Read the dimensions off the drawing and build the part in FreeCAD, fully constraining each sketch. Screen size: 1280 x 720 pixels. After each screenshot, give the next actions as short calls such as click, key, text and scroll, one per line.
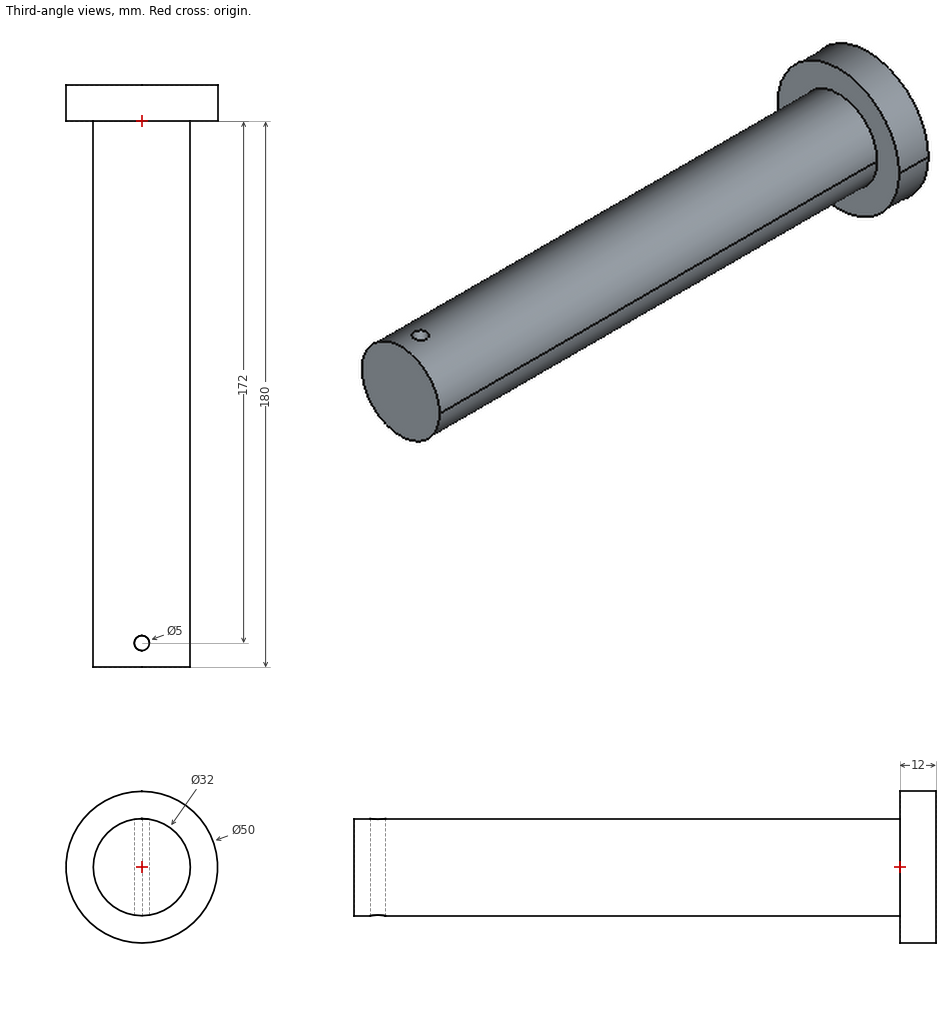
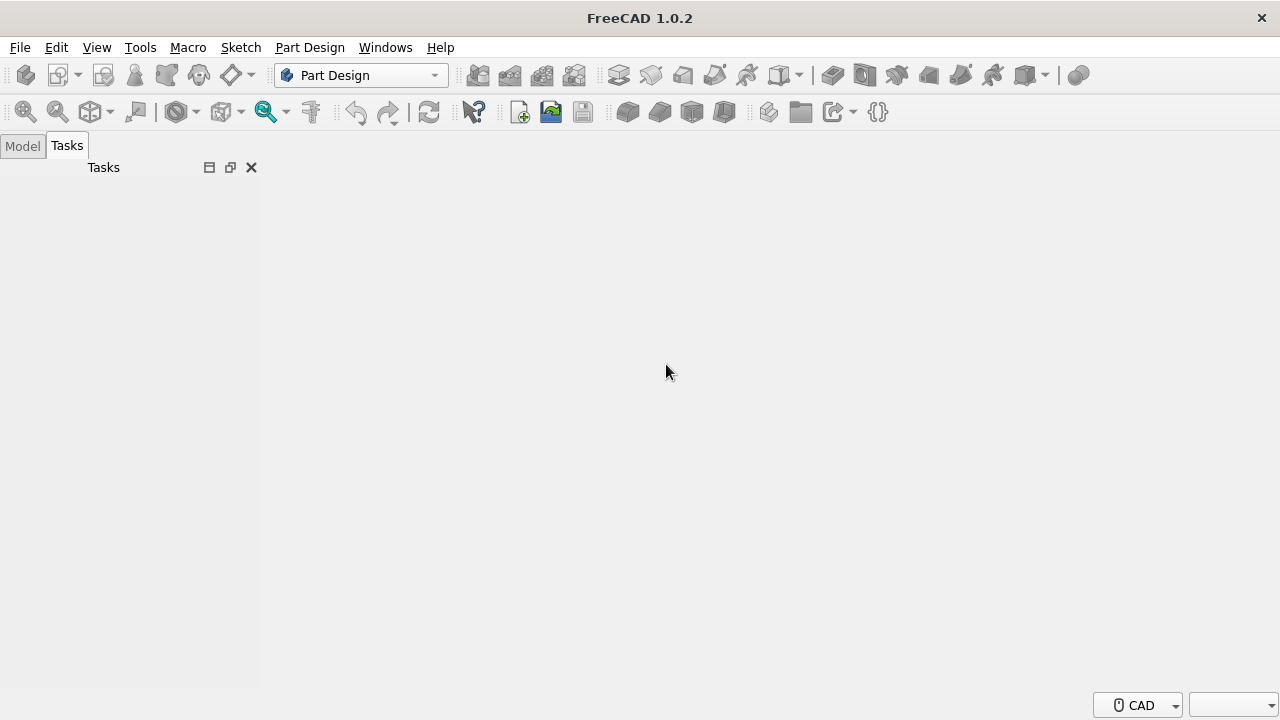
click(520, 112)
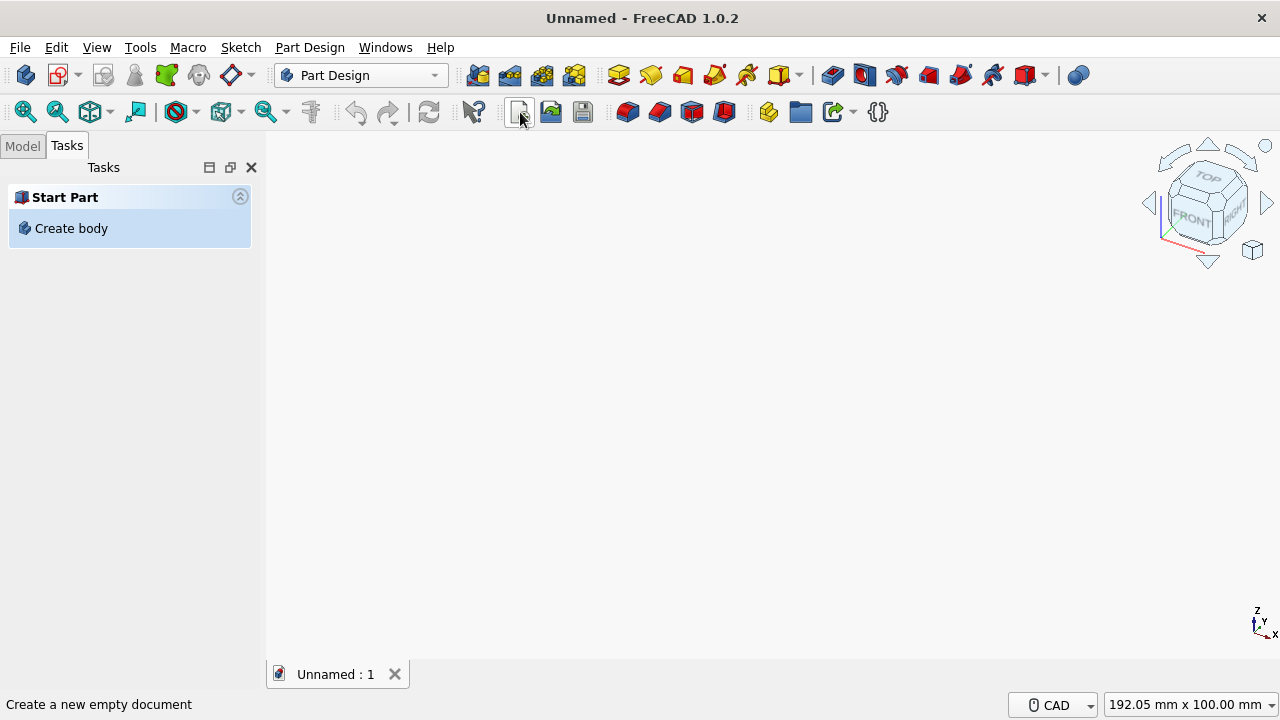
click(58, 76)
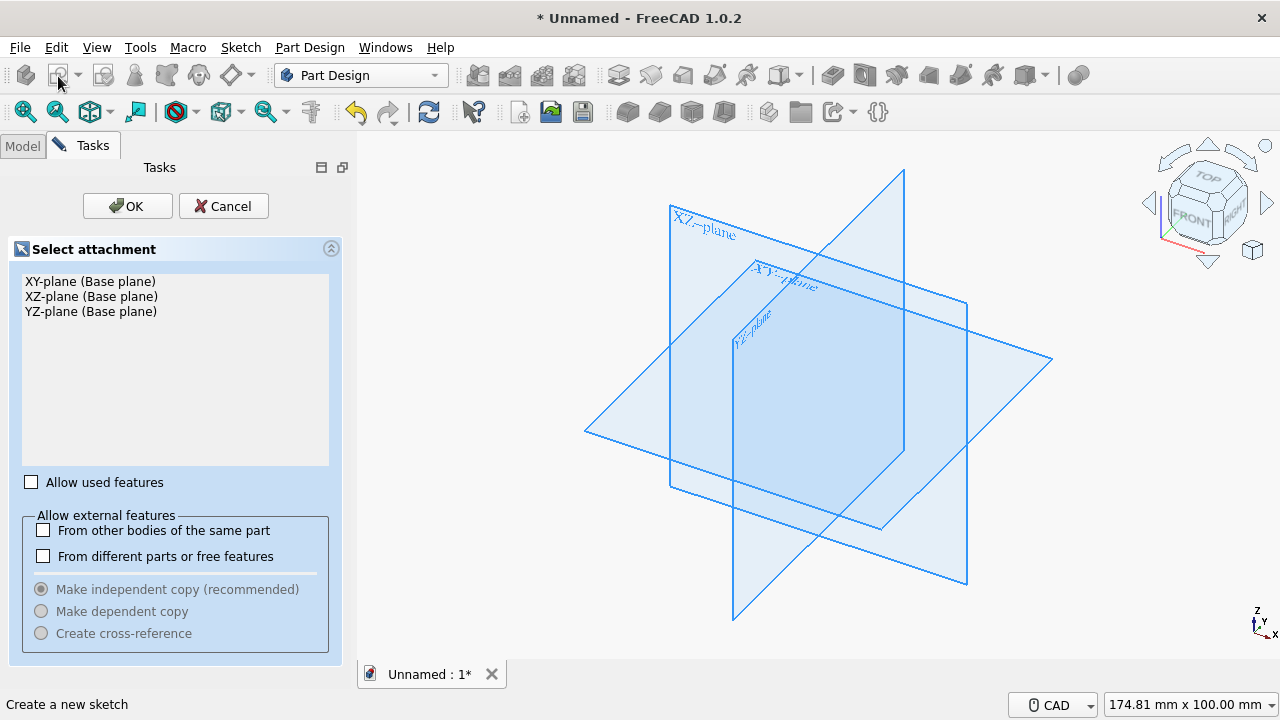
click(82, 296)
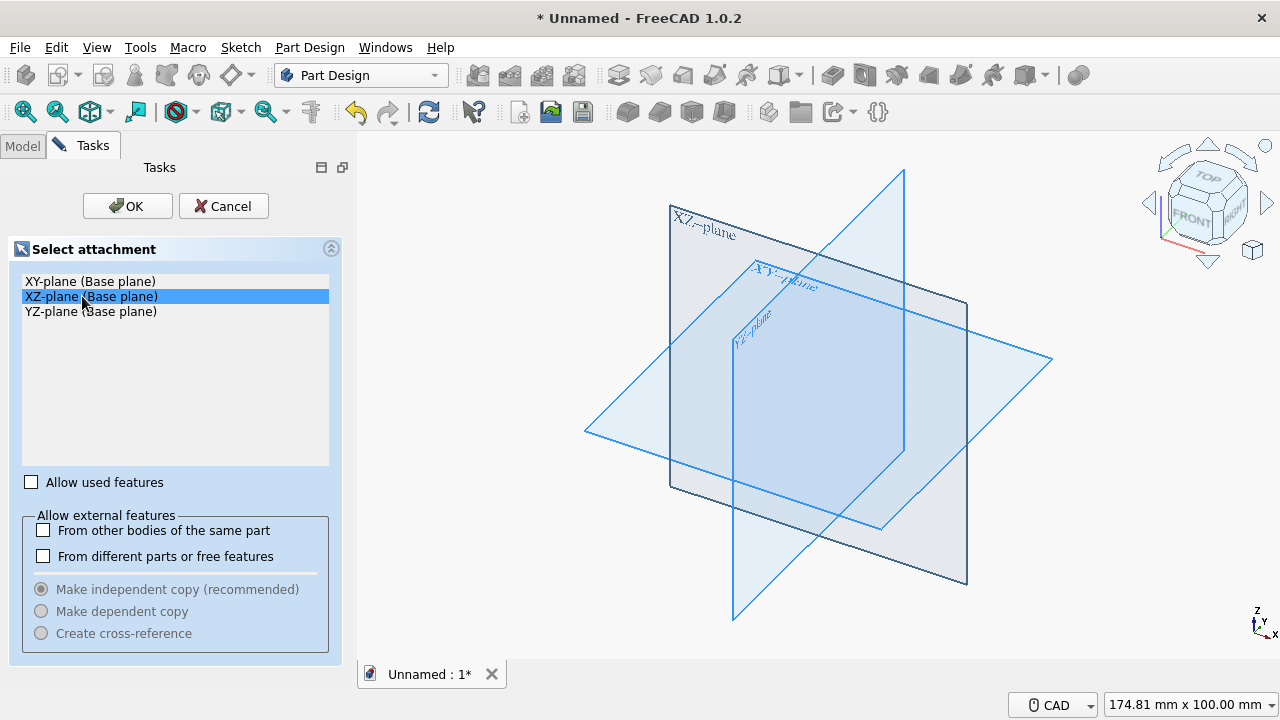
click(128, 206)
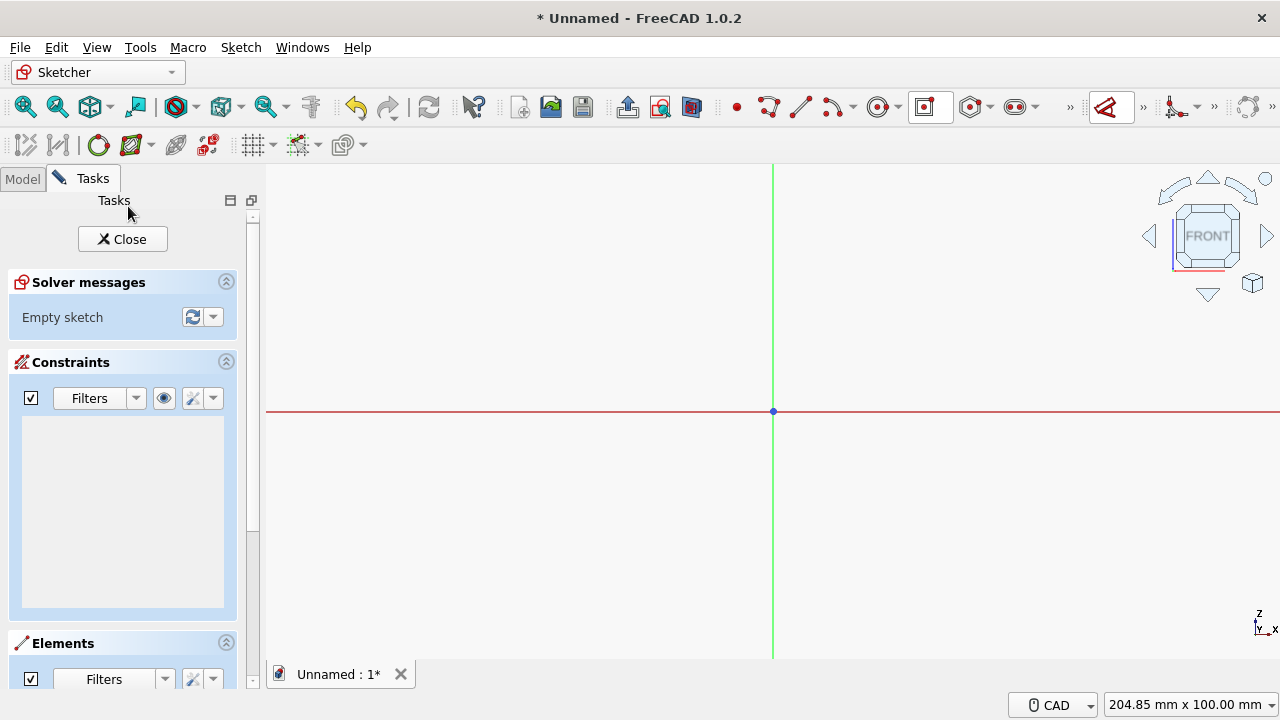
click(878, 108)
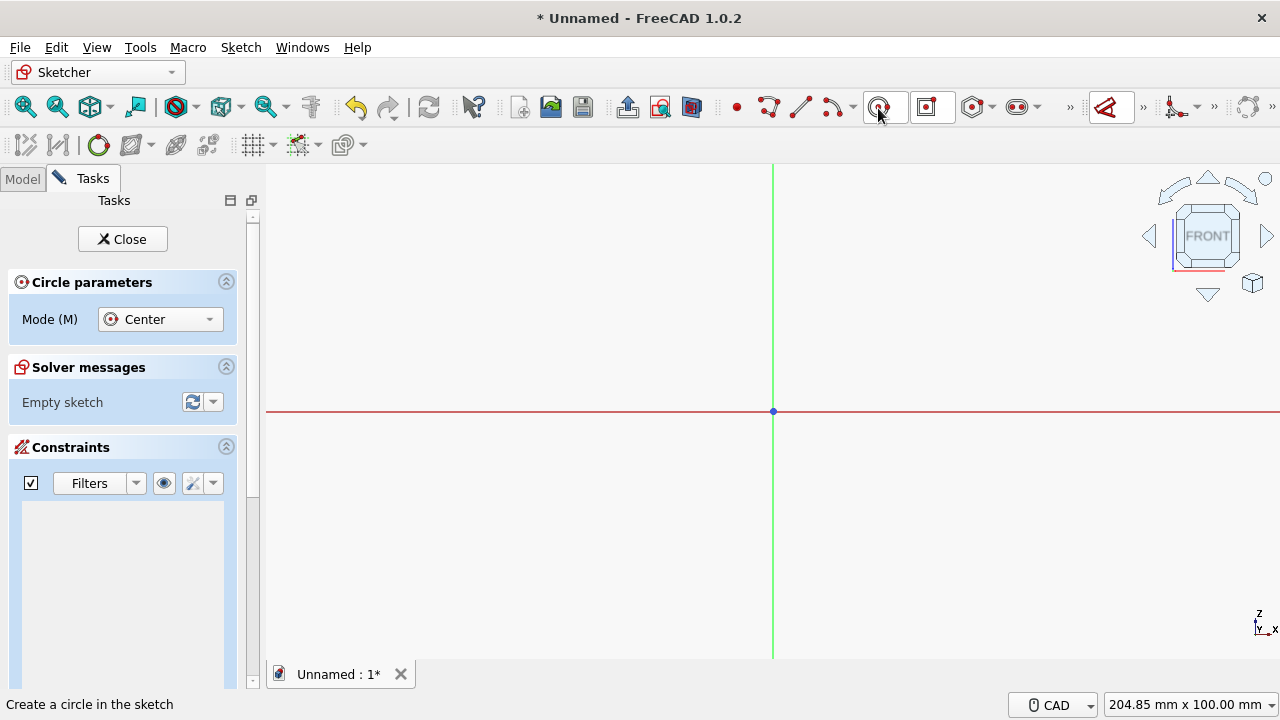
click(773, 412)
move(861, 324)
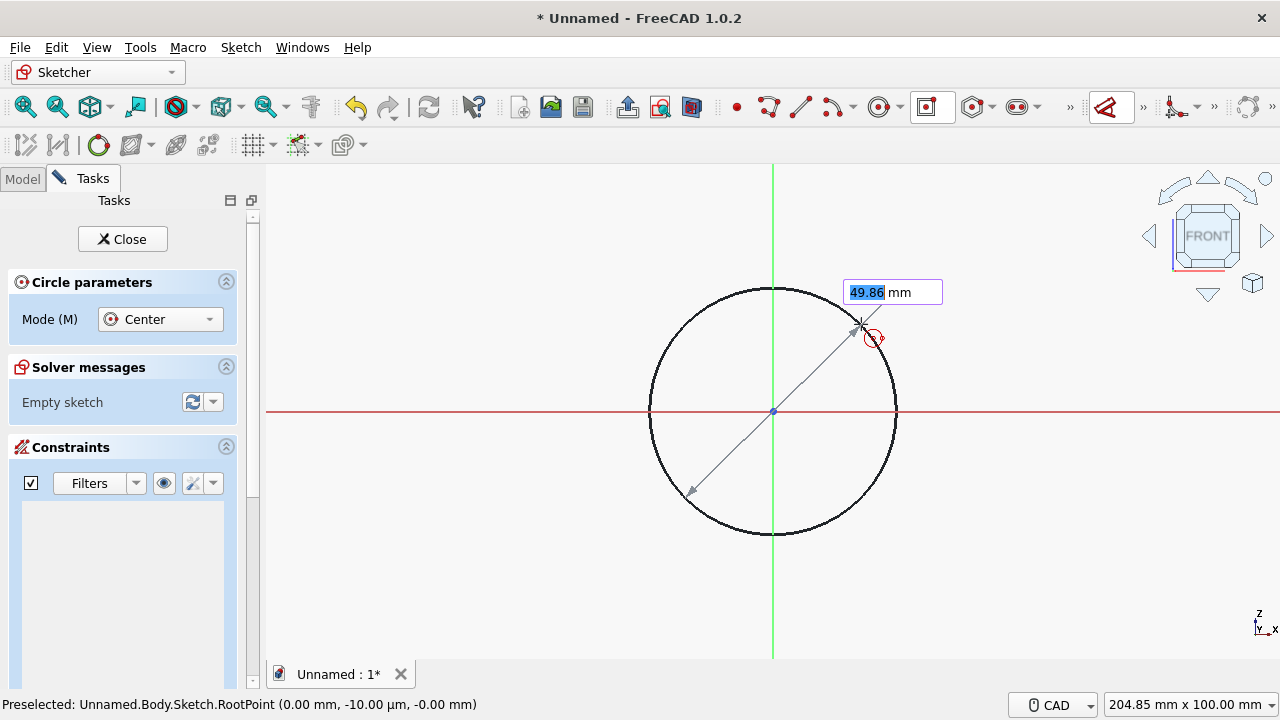
text(50)
key(Return)
key(Escape)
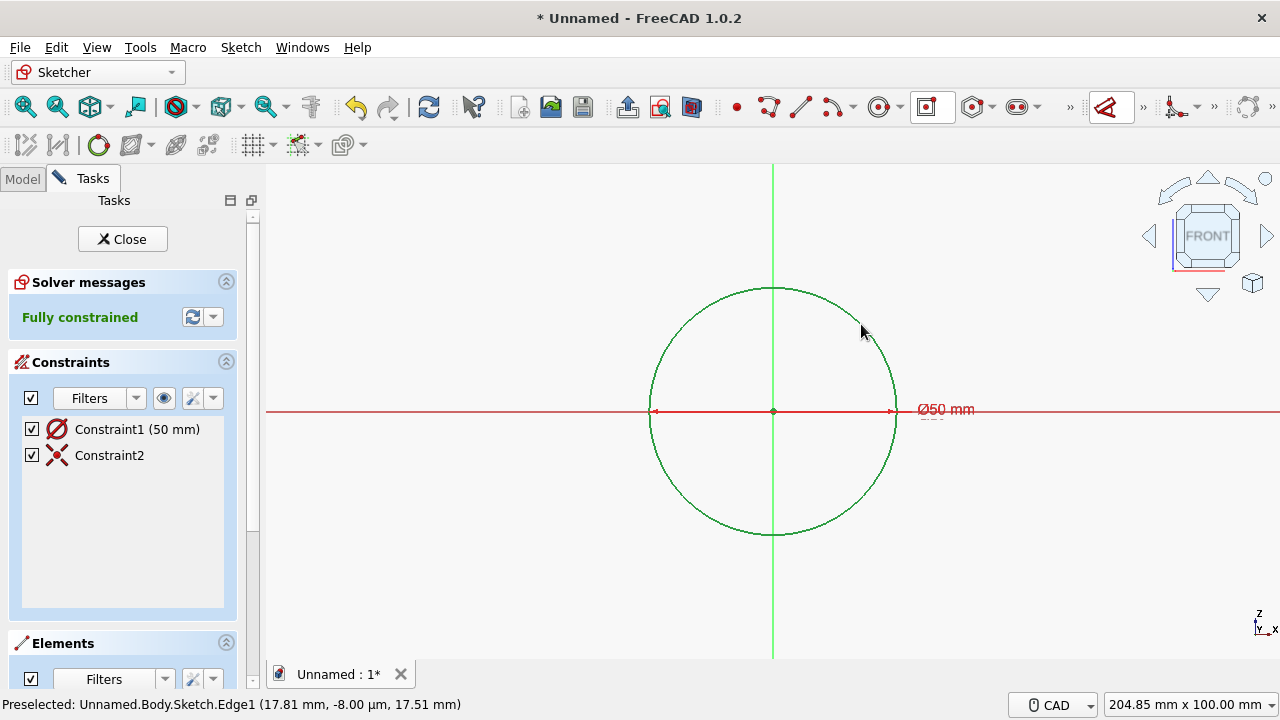
click(123, 239)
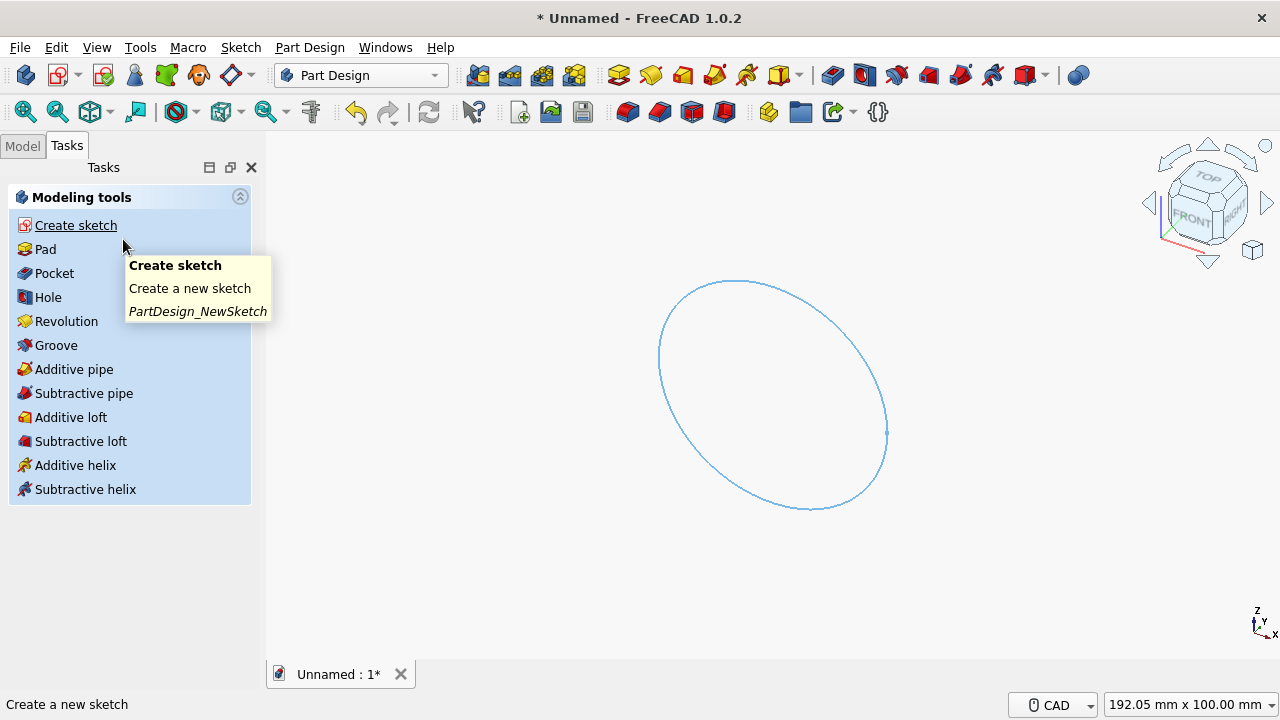
click(620, 76)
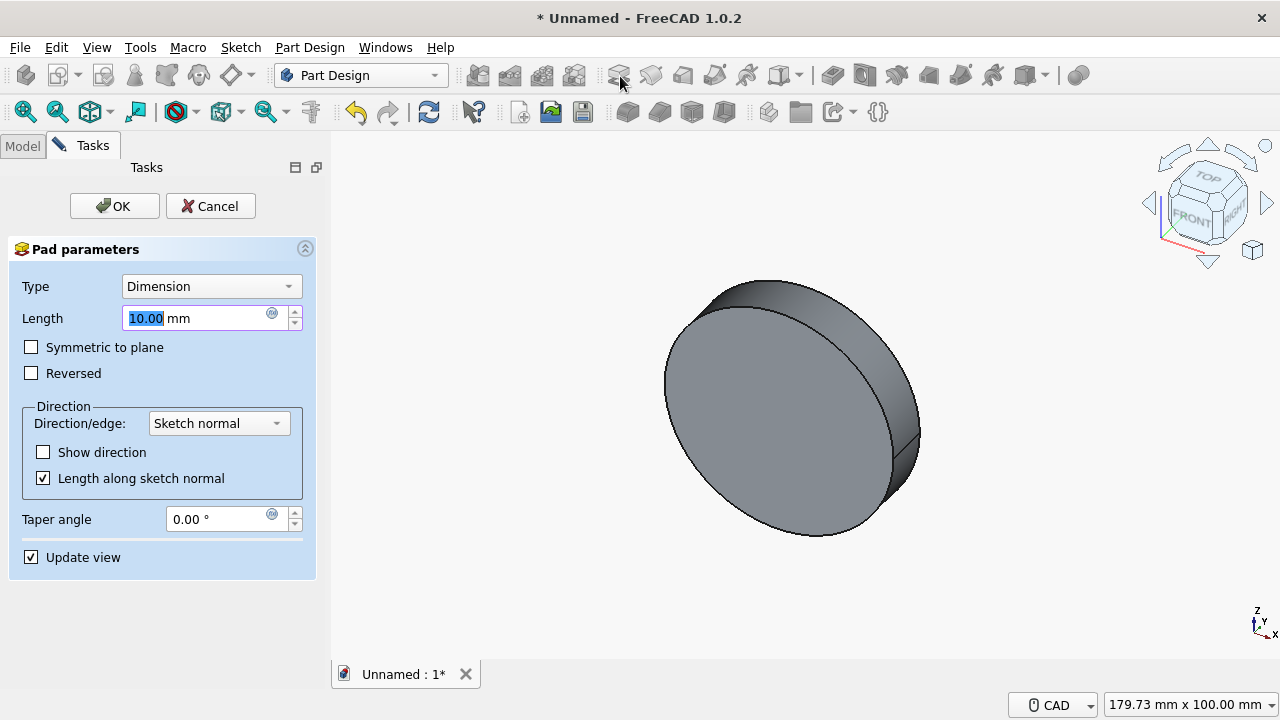
text(12)
key(Tab)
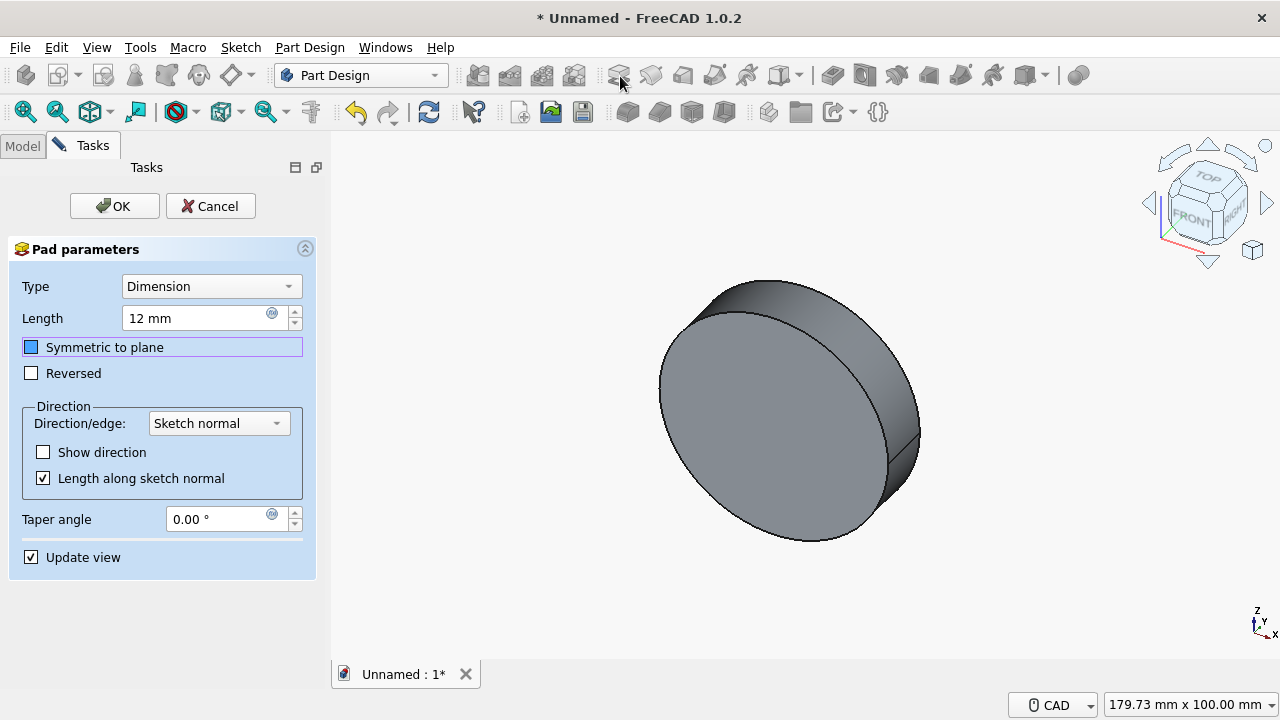
click(30, 373)